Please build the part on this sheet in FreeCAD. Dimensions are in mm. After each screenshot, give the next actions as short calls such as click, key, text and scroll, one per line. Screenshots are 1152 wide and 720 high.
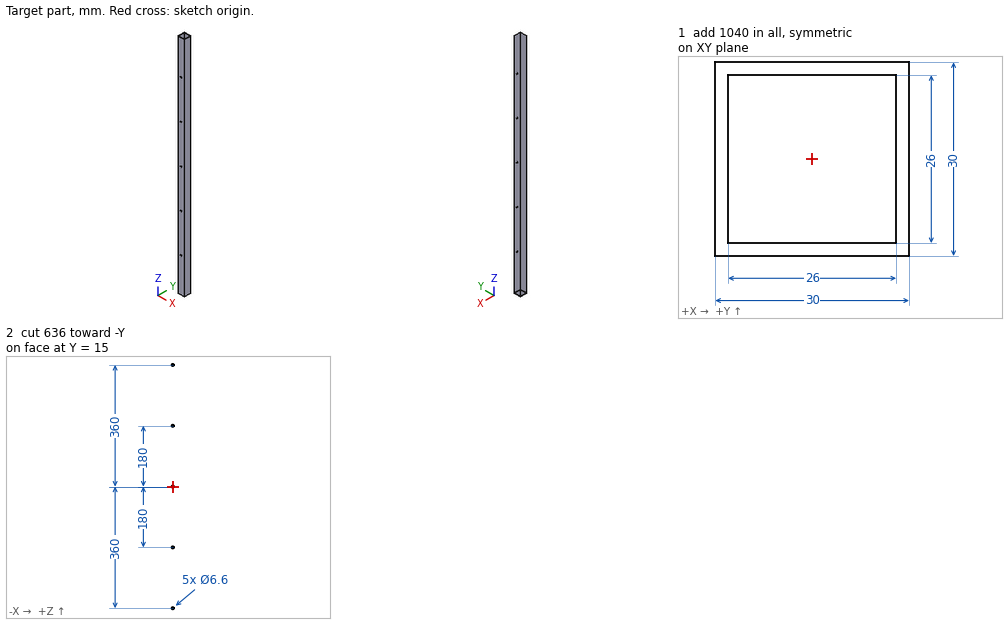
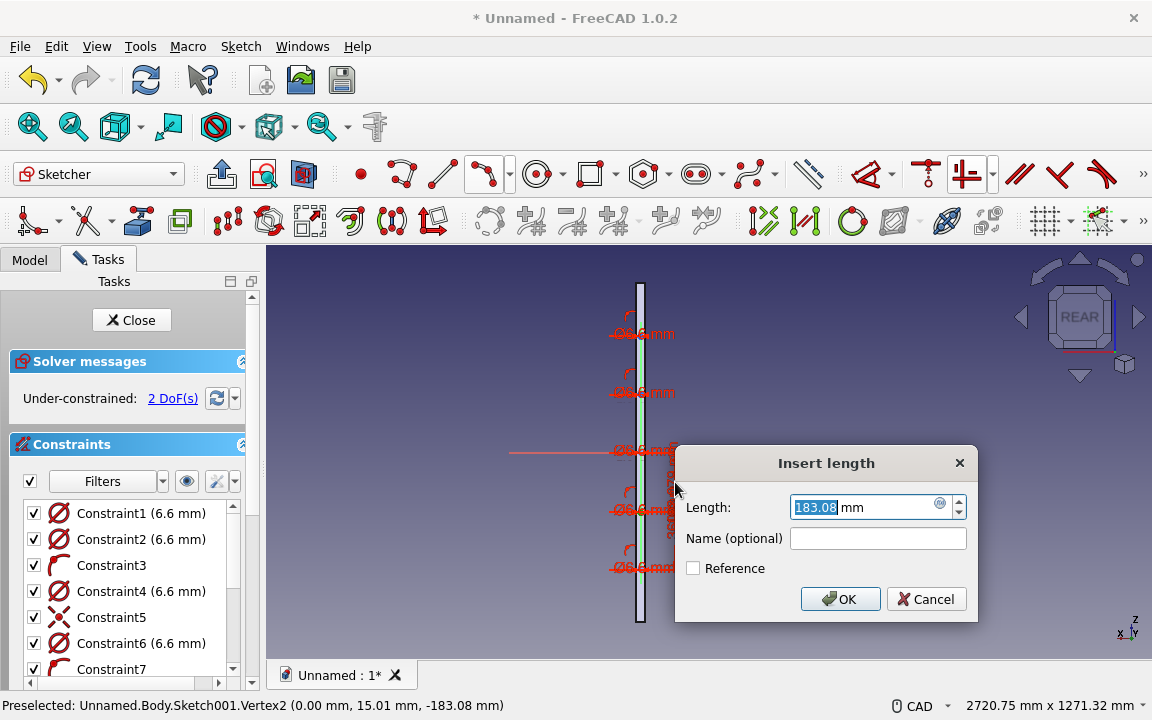
text(180)
key(Return)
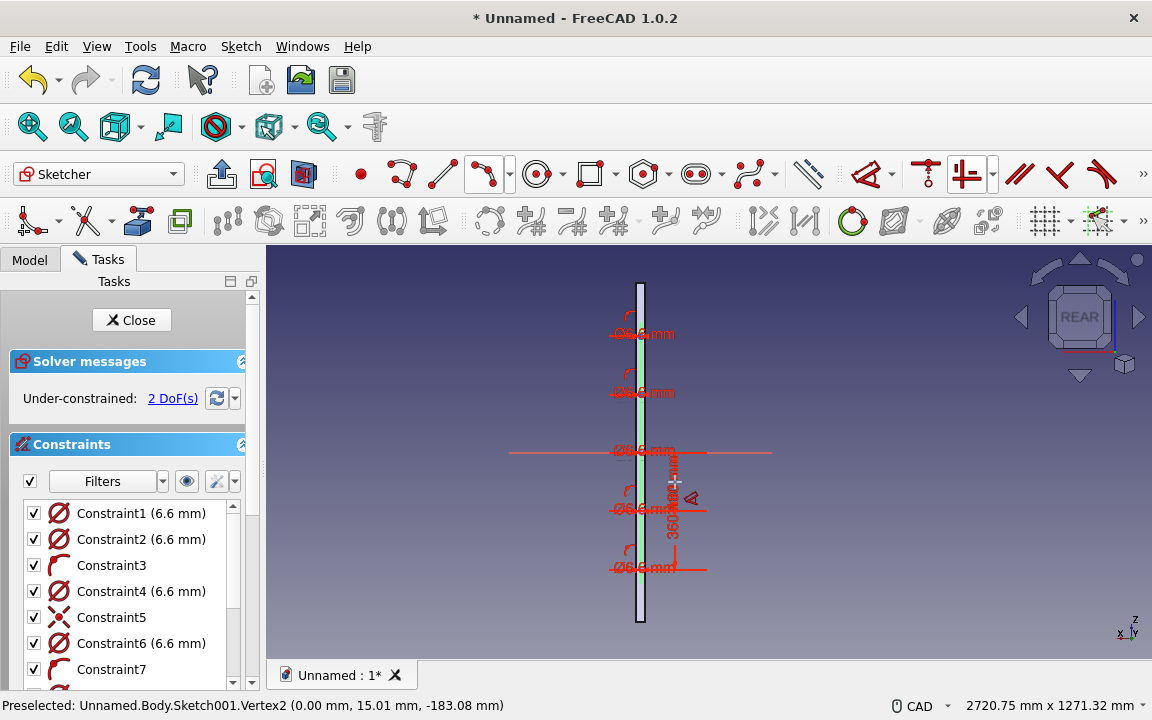
click(641, 395)
click(675, 424)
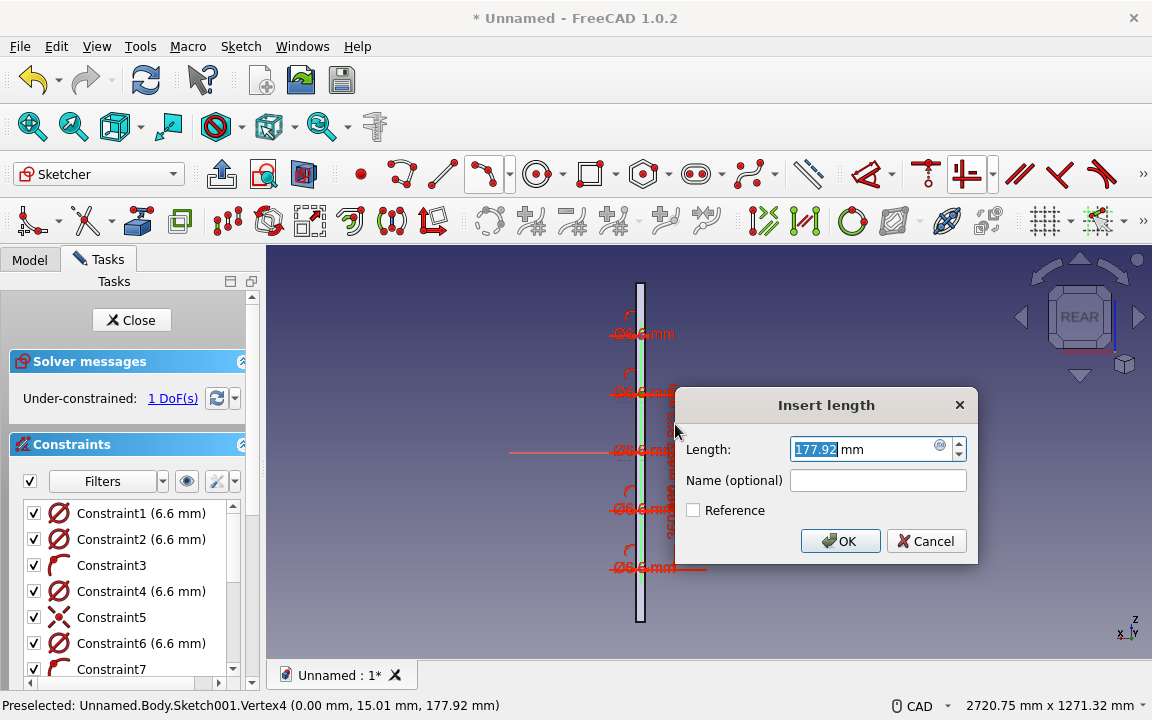
text(180)
key(Return)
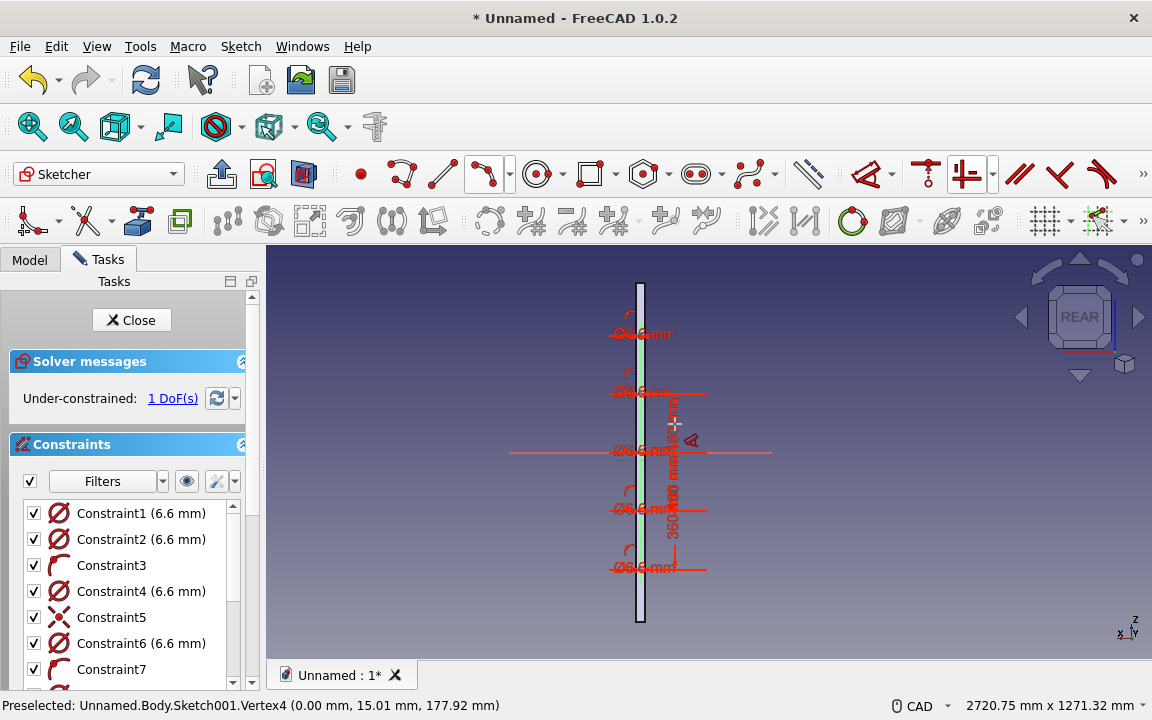
click(641, 336)
click(675, 394)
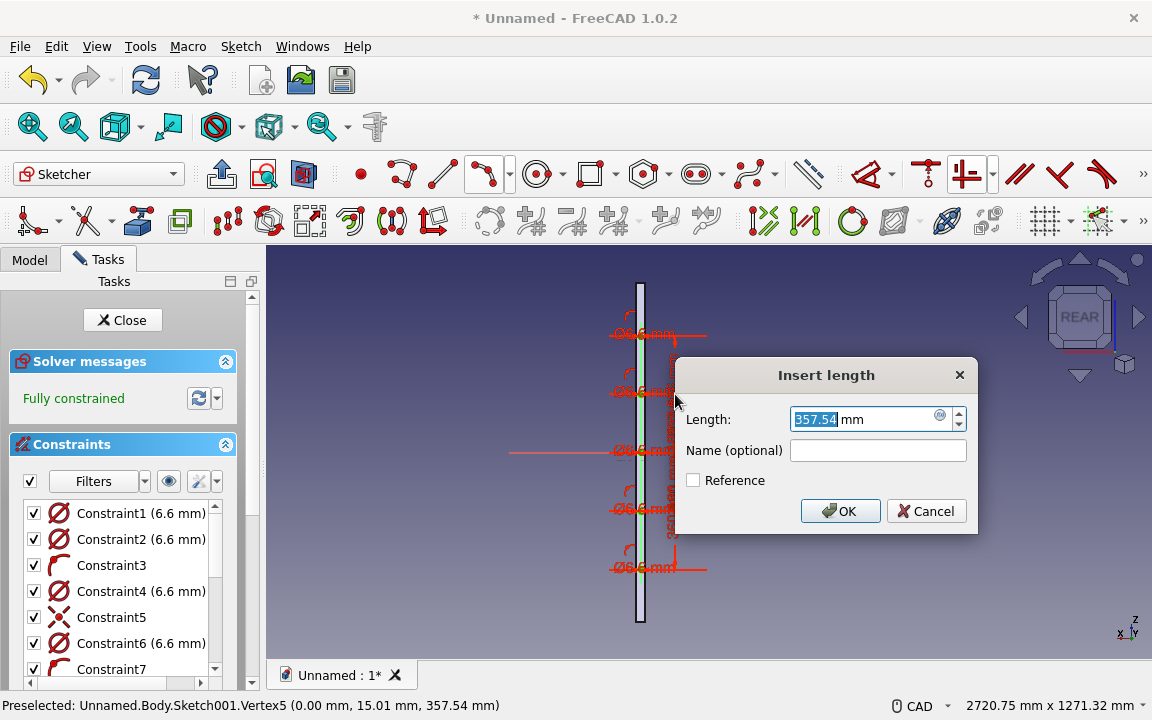
text(360)
key(Return)
key(Escape)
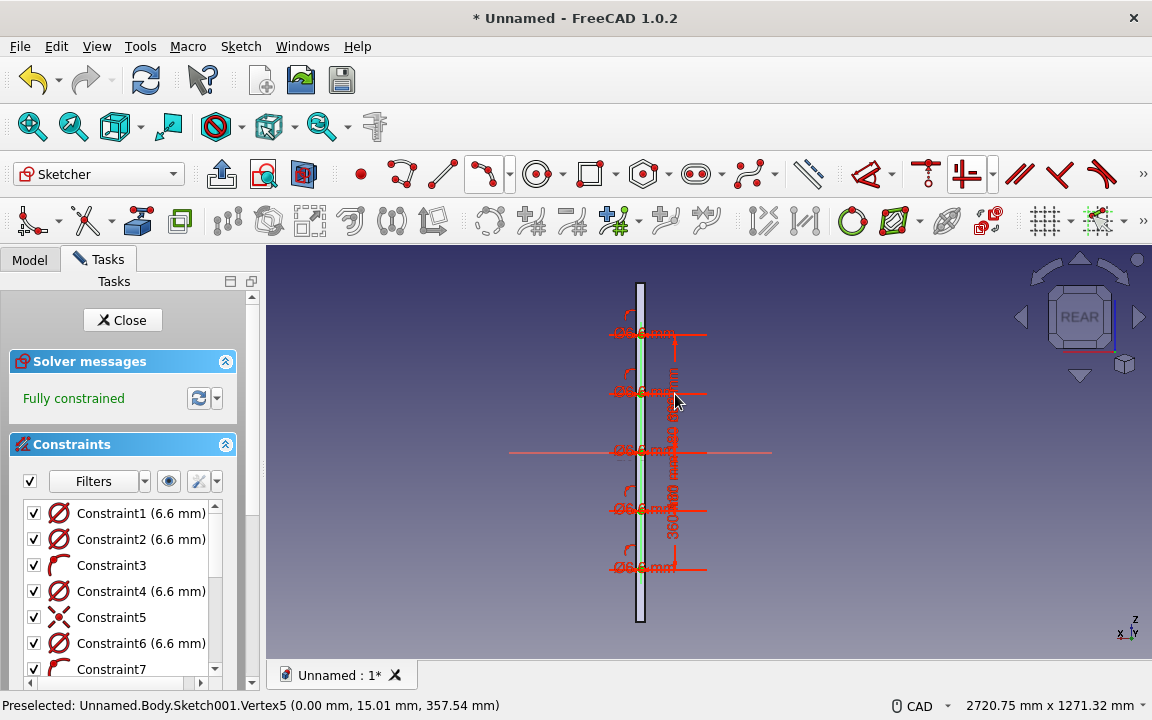
click(123, 320)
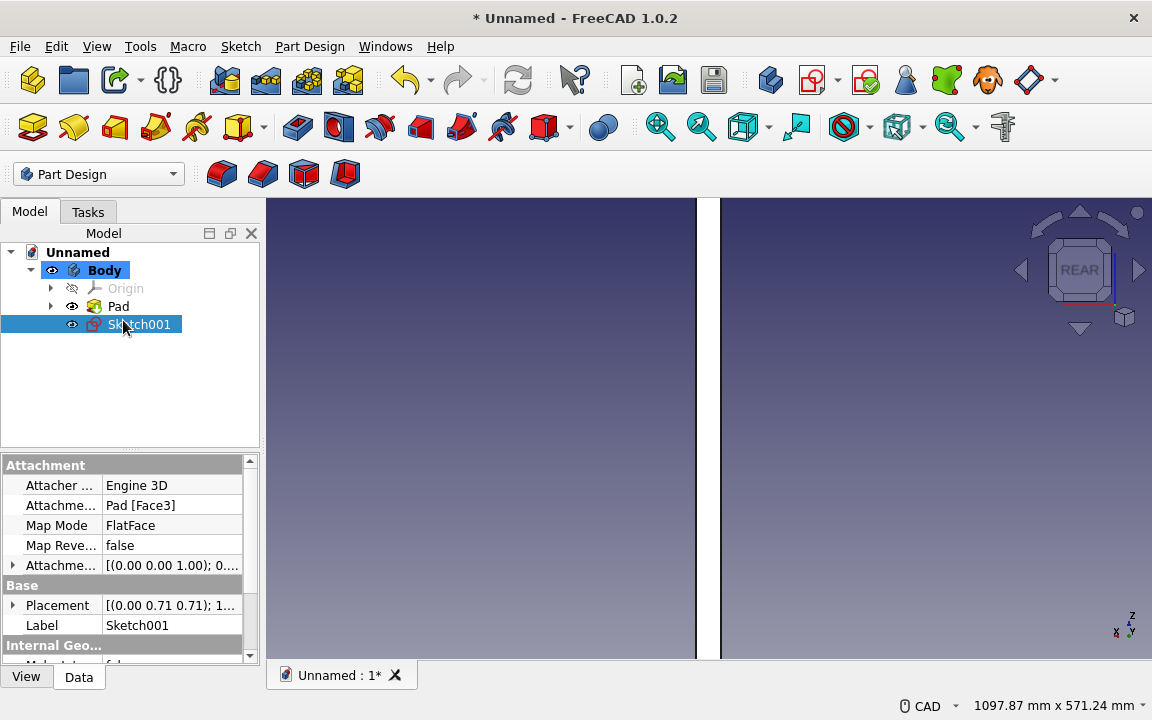
click(298, 128)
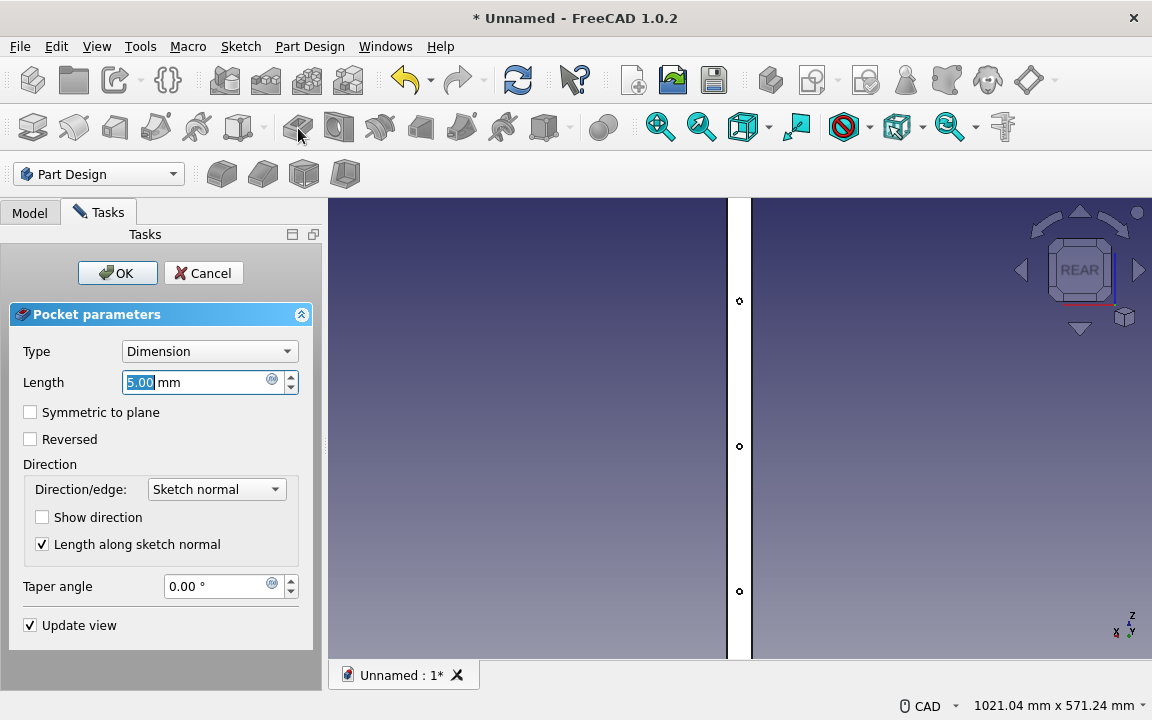
text(636)
key(Tab)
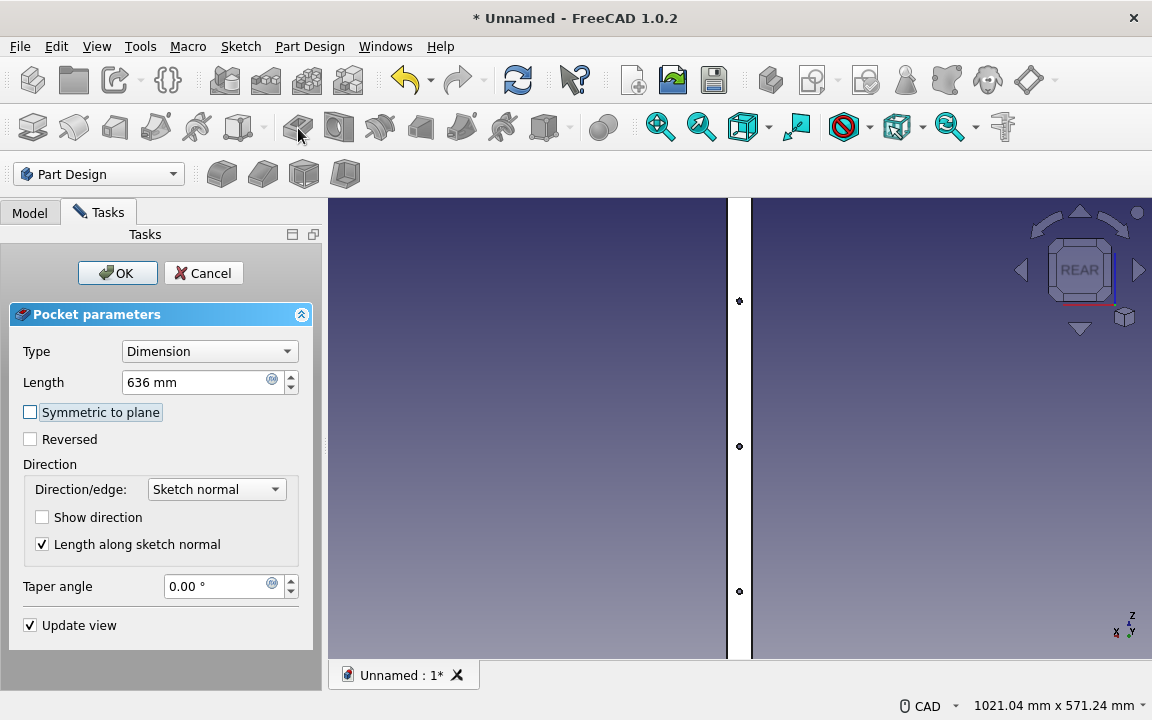
click(118, 273)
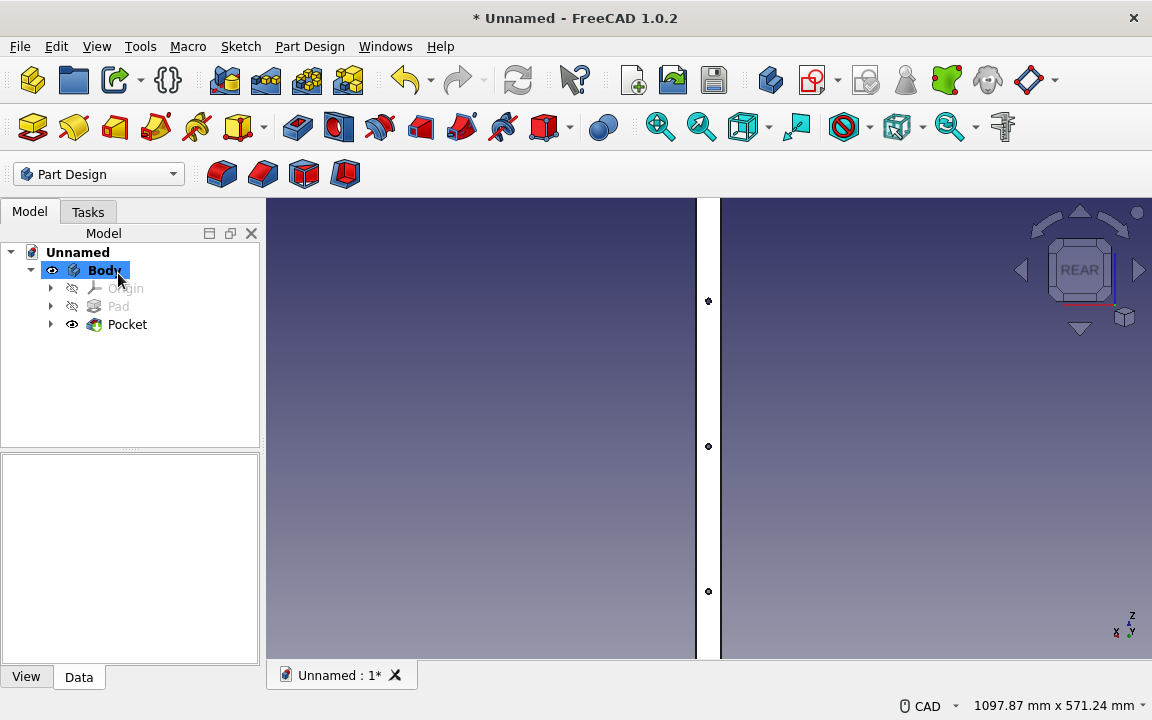
key(0)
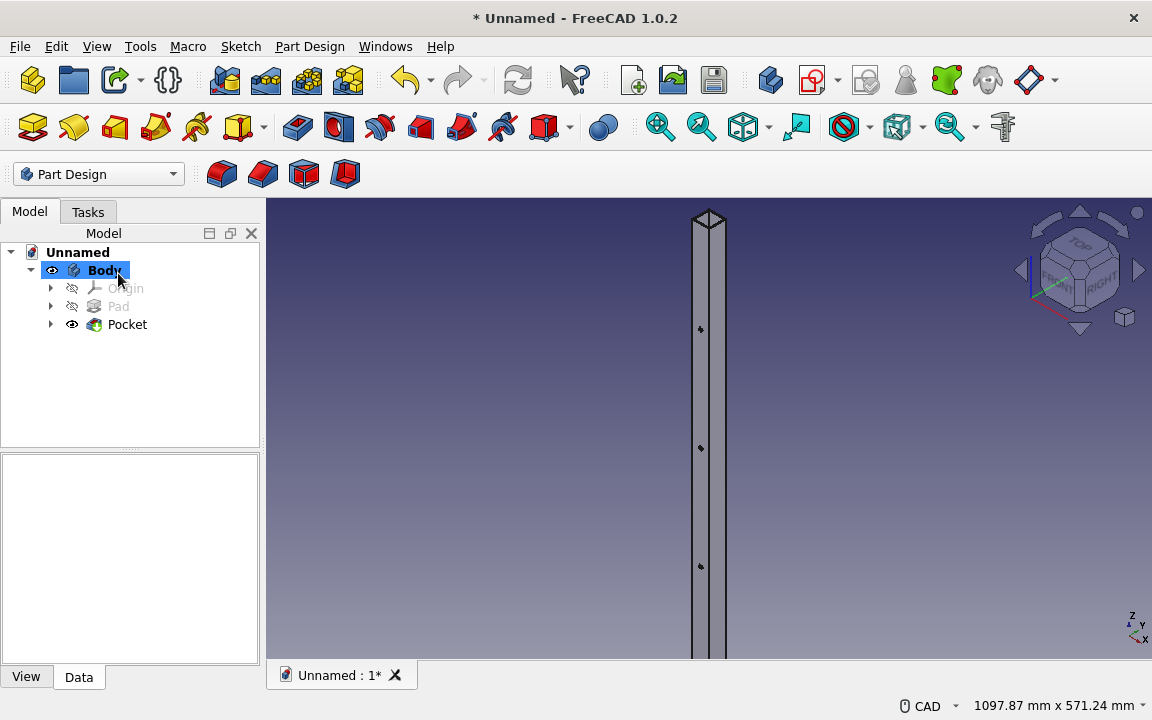
key(v)
key(f)